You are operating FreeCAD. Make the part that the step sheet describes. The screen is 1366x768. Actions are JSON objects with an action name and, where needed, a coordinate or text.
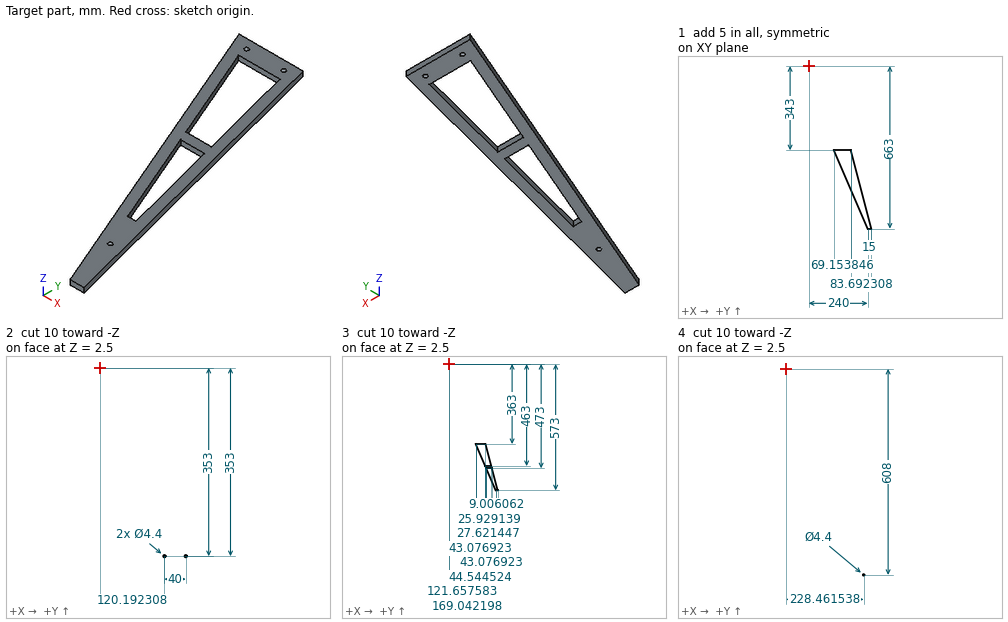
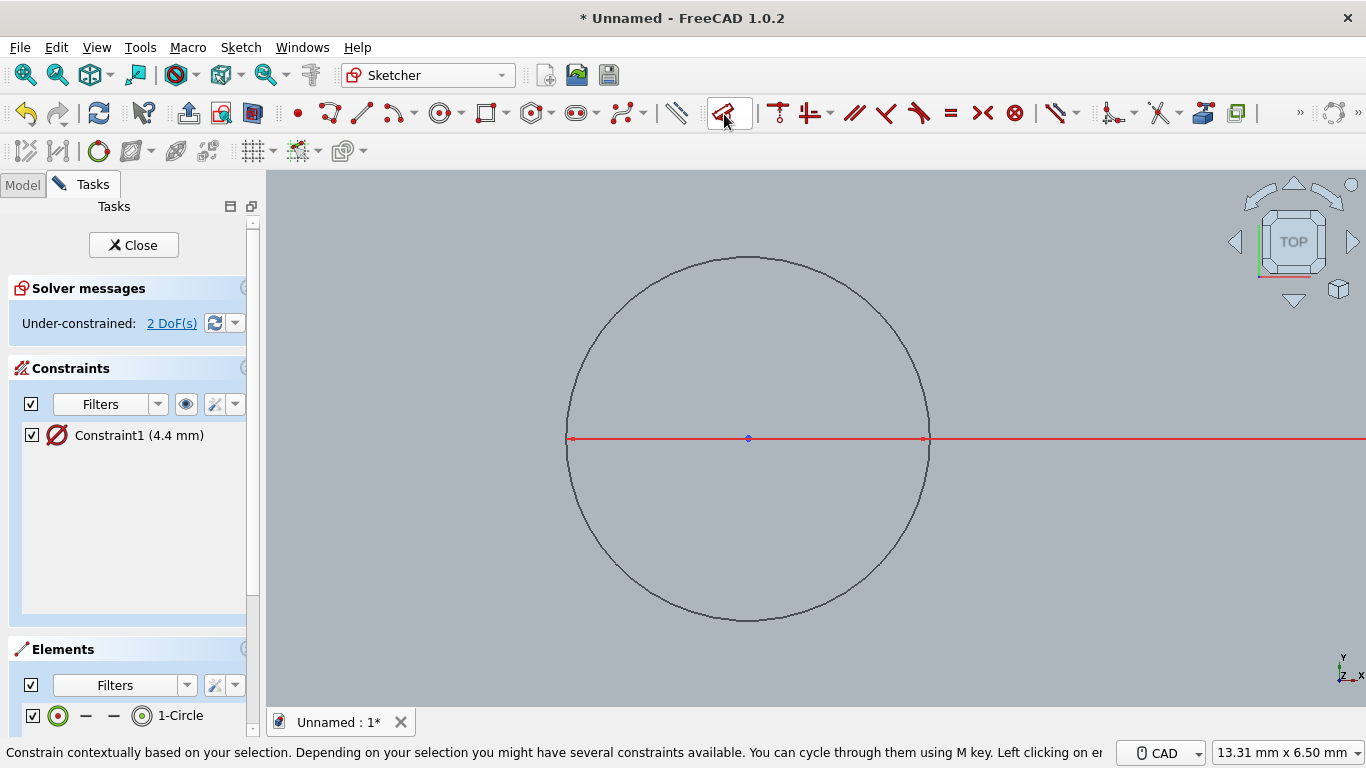
{"action": "left_click", "coordinate": [748, 439]}
{"action": "left_click", "coordinate": [782, 318]}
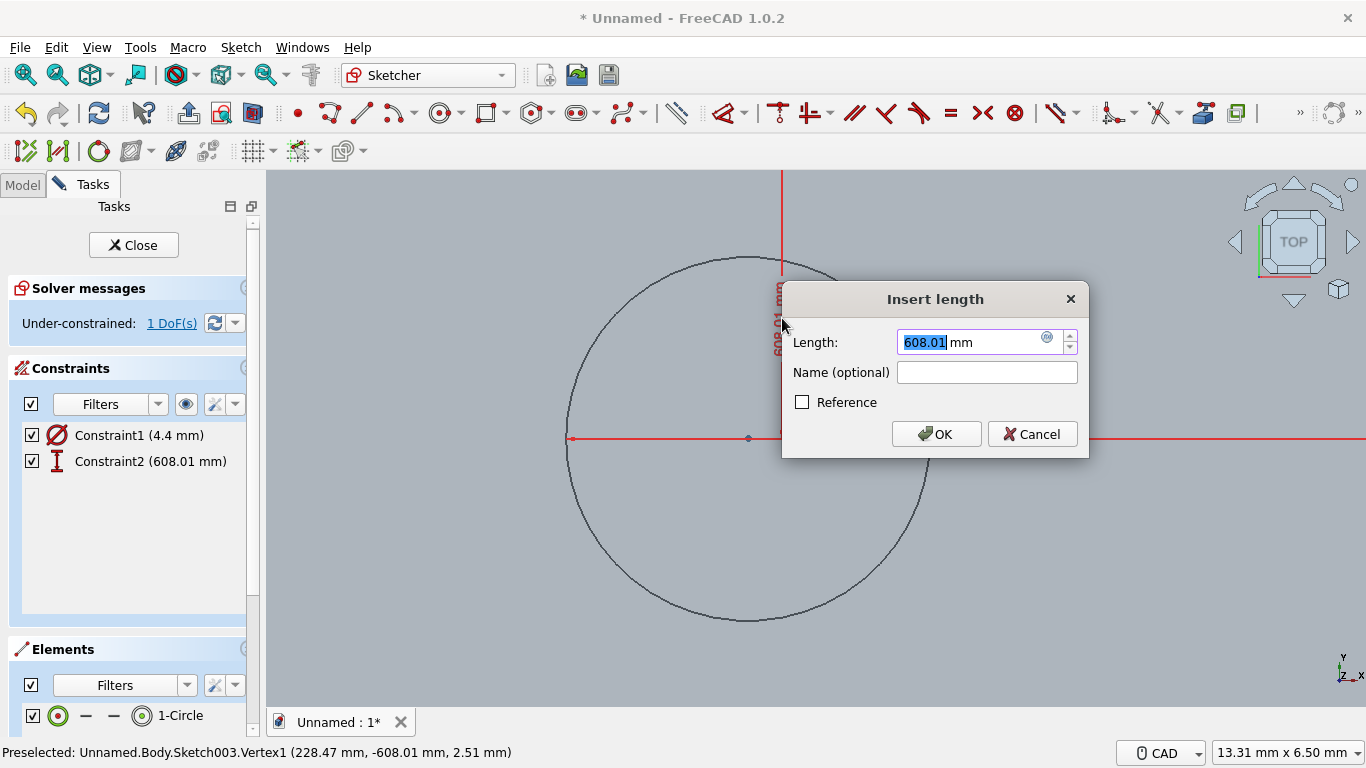
{"action": "type", "text": "608"}
{"action": "key", "text": "Return"}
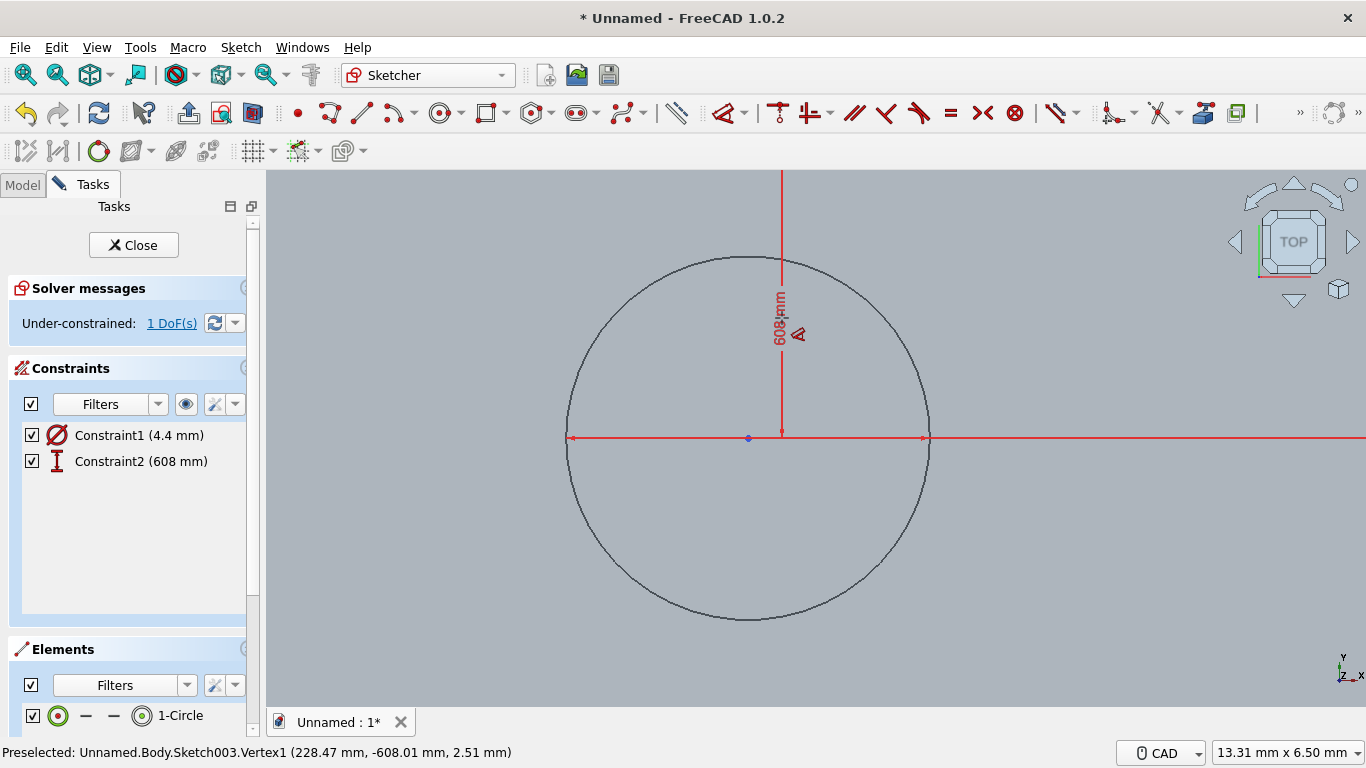
{"action": "left_click", "coordinate": [748, 438]}
{"action": "left_click", "coordinate": [521, 472]}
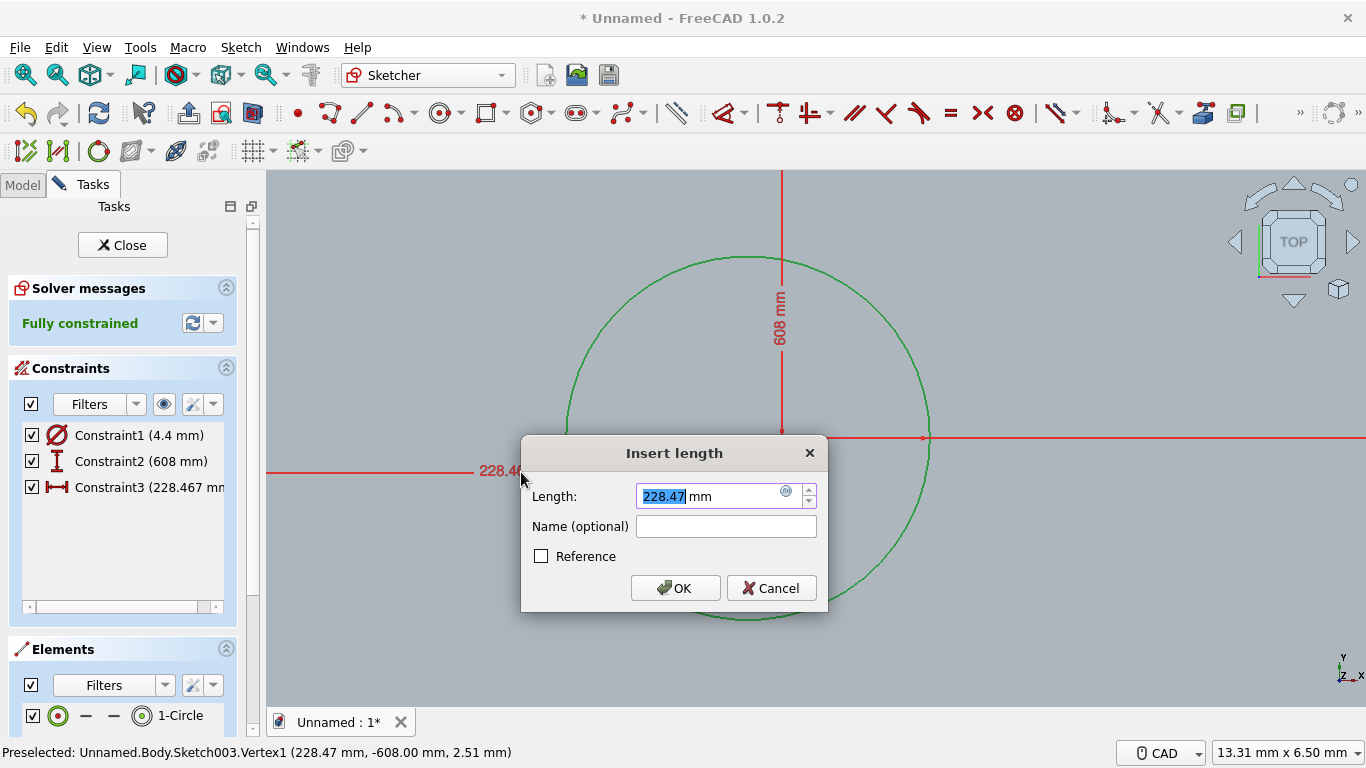
{"action": "type", "text": "228.461538"}
{"action": "key", "text": "Return"}
{"action": "key", "text": "Escape"}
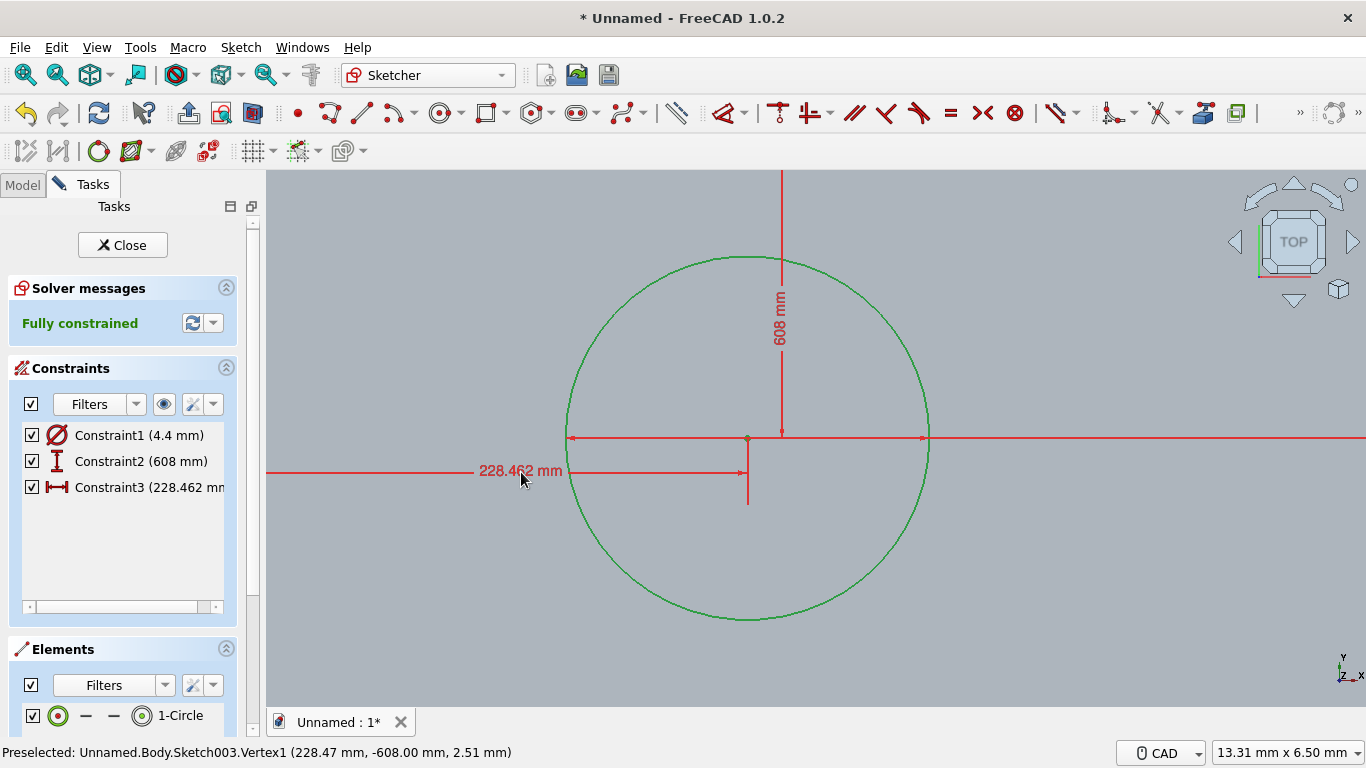
{"action": "left_click", "coordinate": [123, 245]}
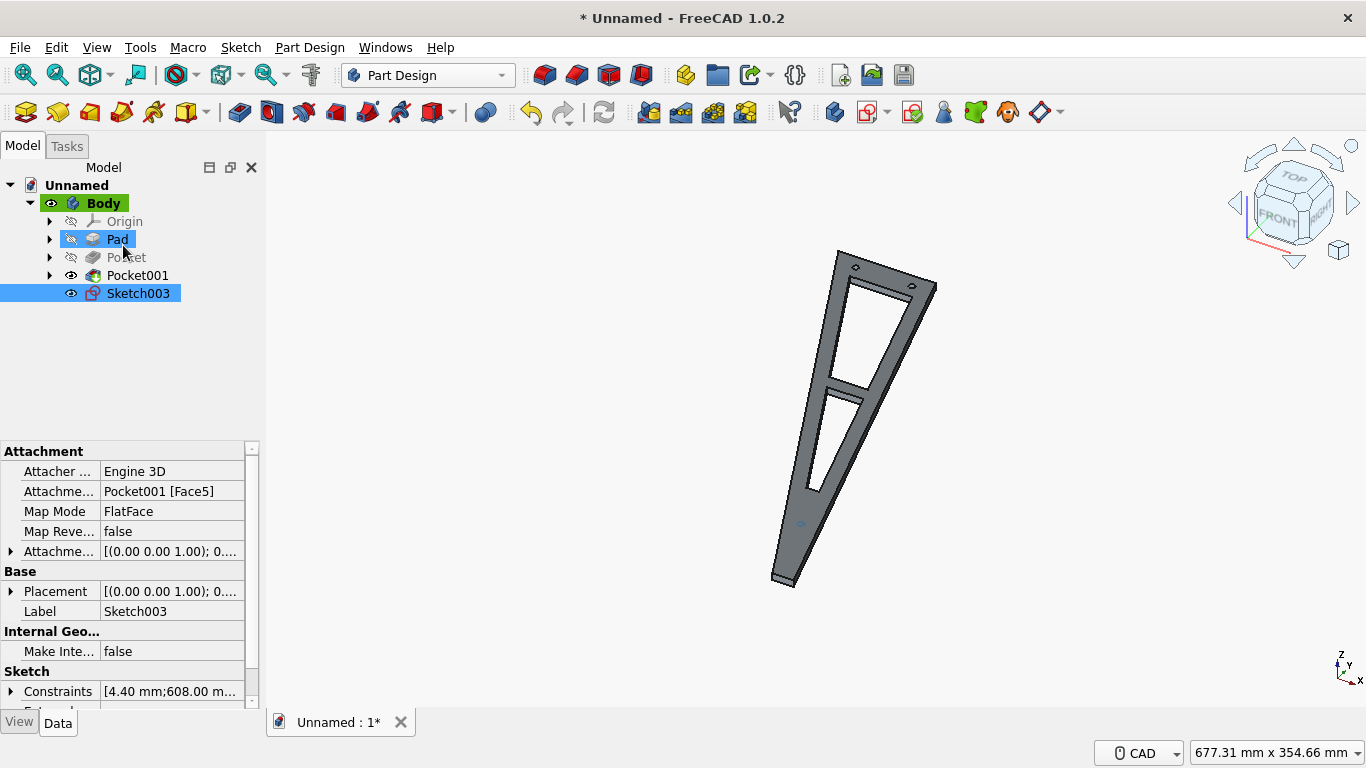
{"action": "left_click", "coordinate": [240, 112]}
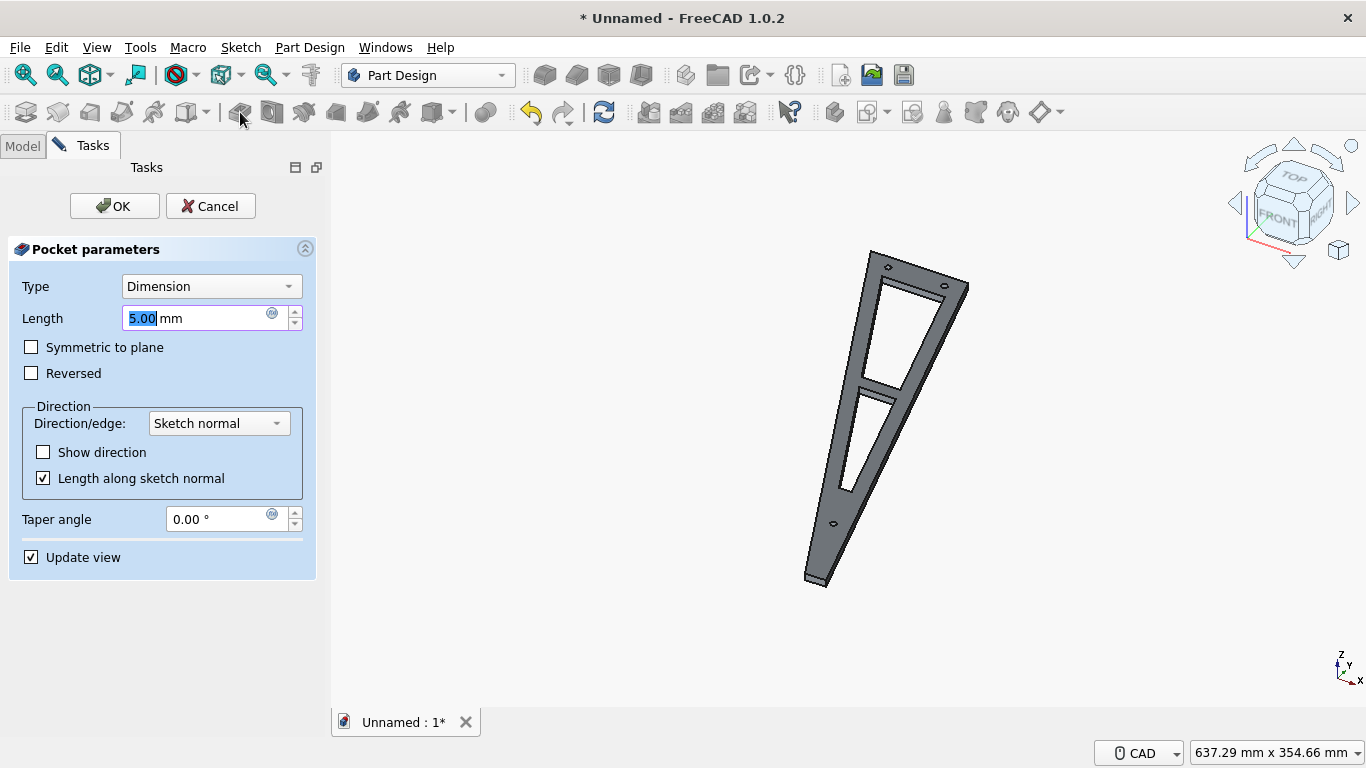
{"action": "type", "text": "10"}
{"action": "key", "text": "Tab"}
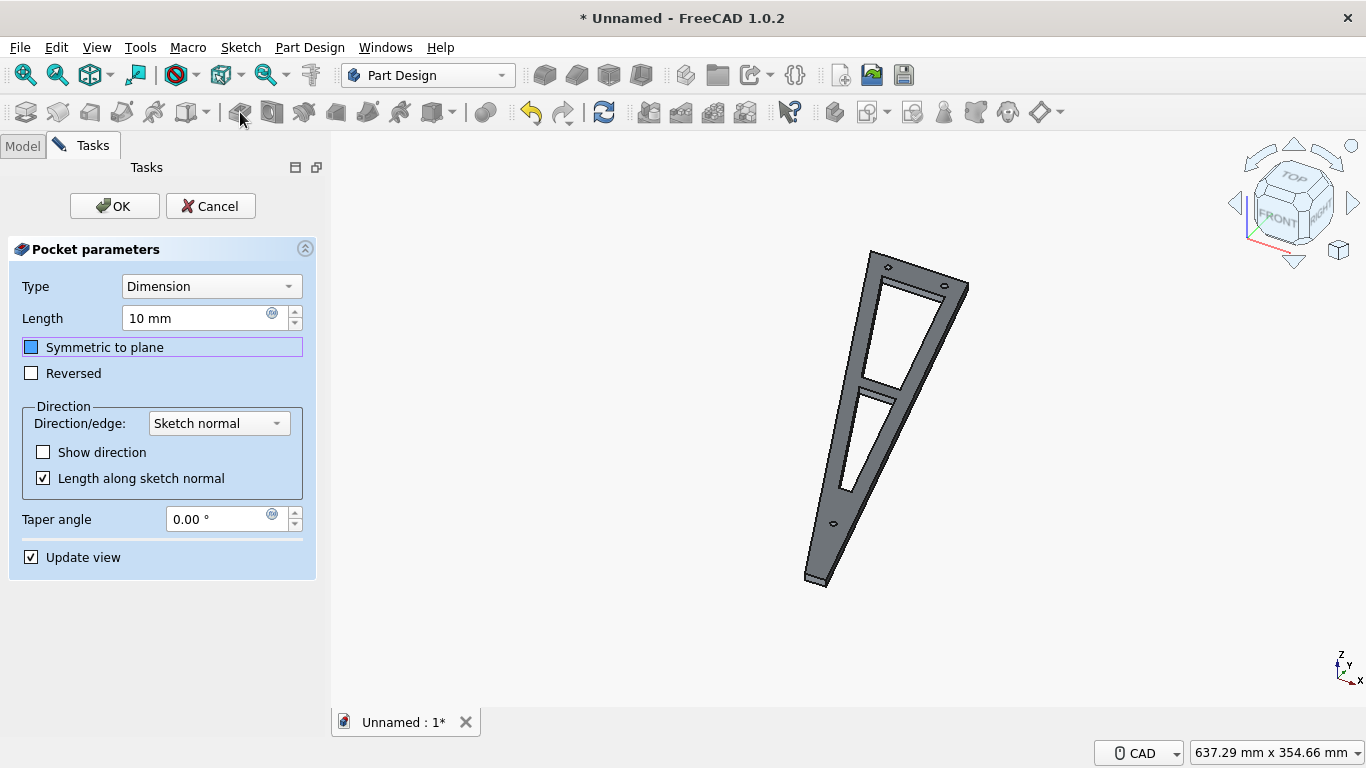
{"action": "left_click", "coordinate": [115, 206]}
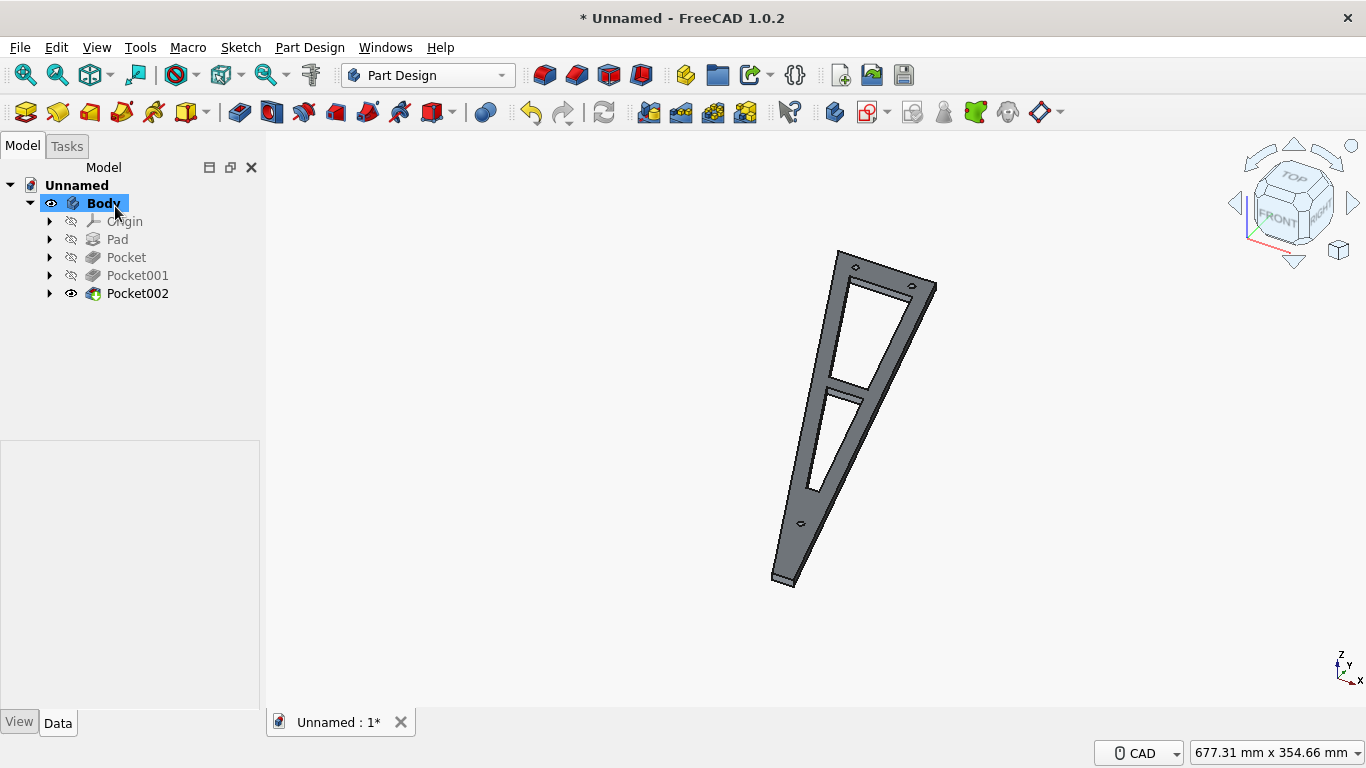
{"action": "key", "text": "0"}